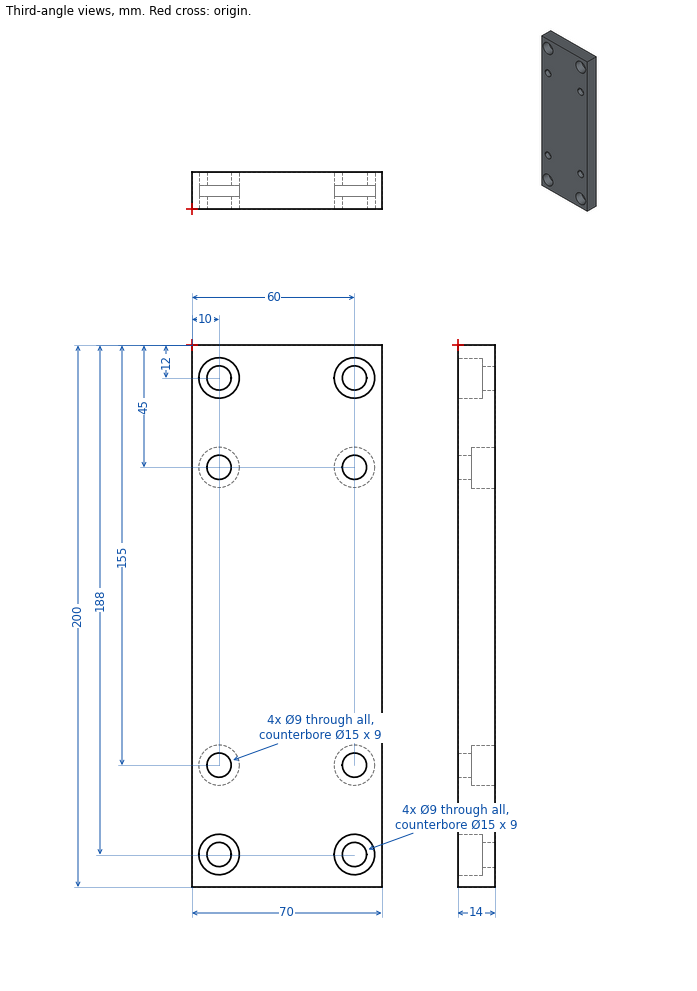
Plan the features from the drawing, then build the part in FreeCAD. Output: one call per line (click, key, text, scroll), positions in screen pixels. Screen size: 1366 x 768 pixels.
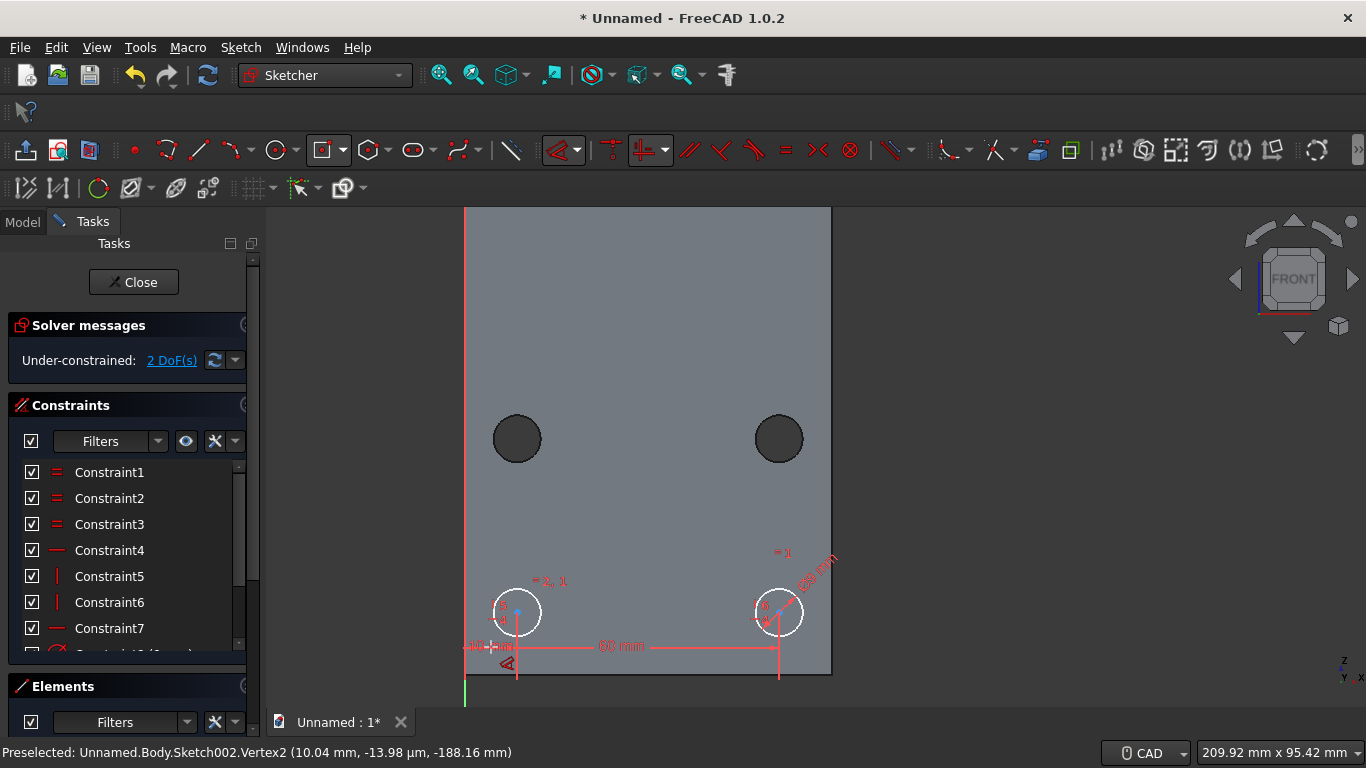
scroll(797, 598, down, 6)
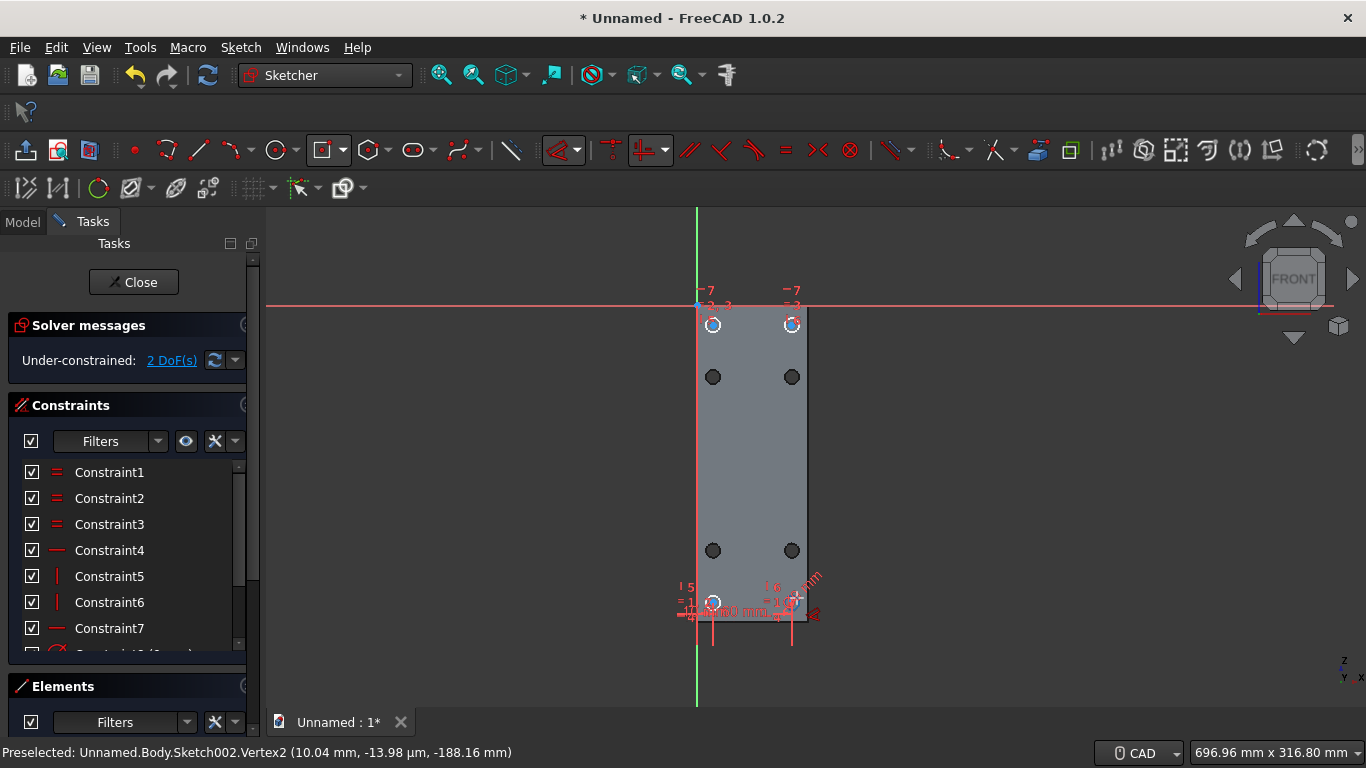
scroll(713, 325, up, 4)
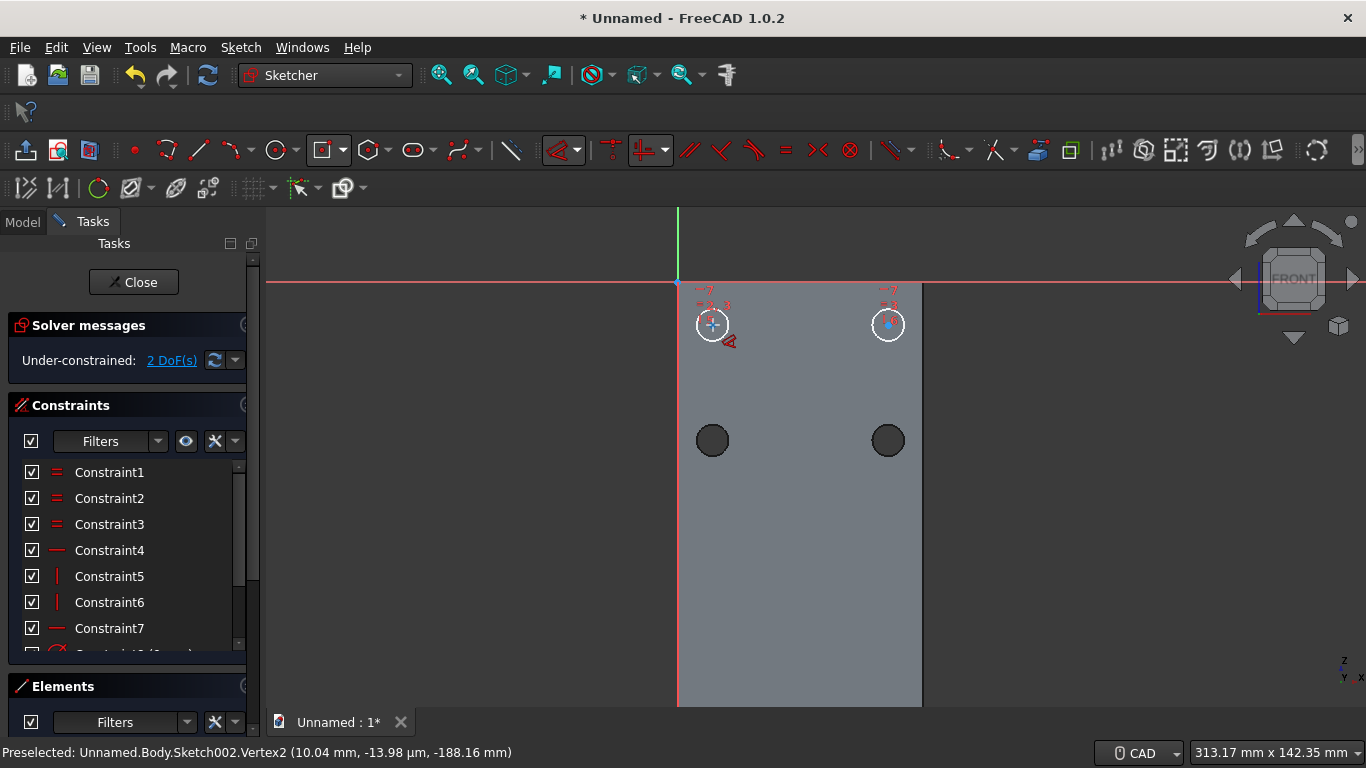
click(713, 325)
click(644, 304)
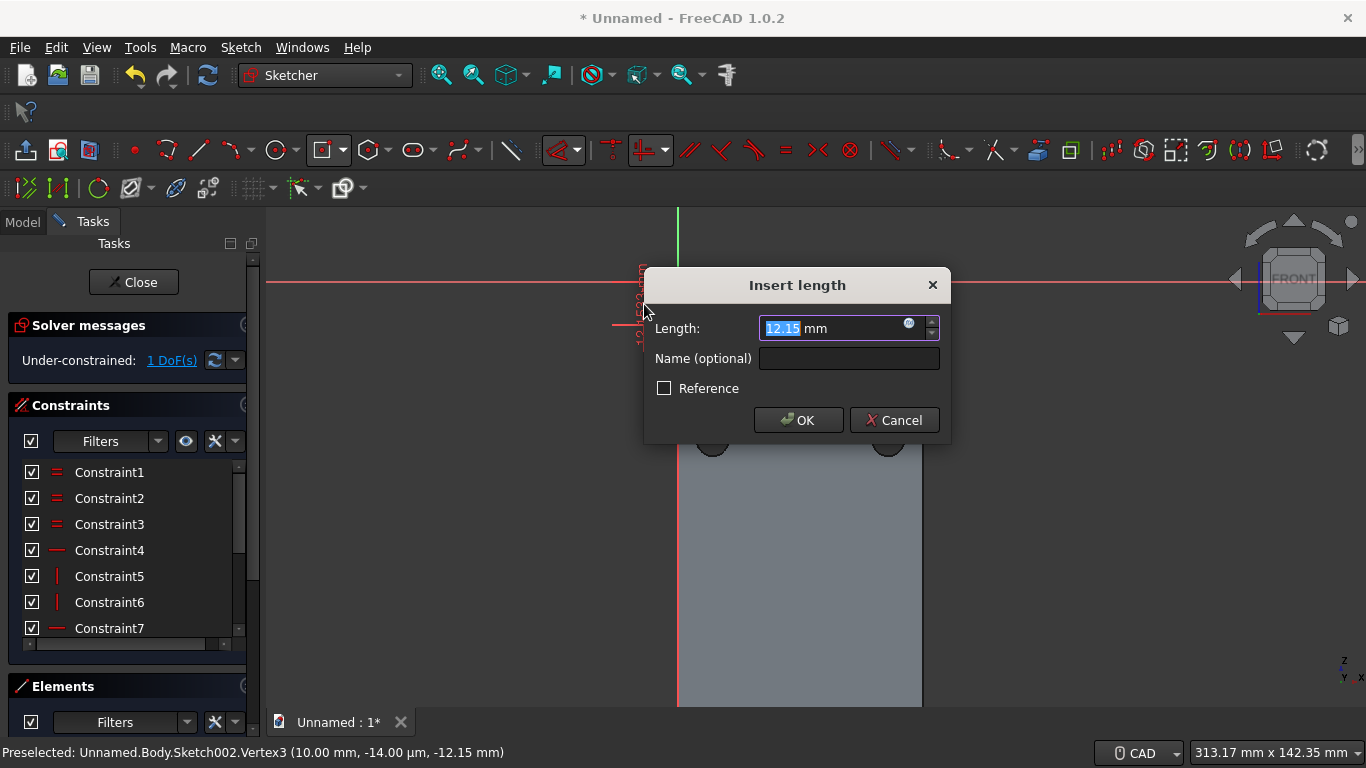
text(12)
key(Return)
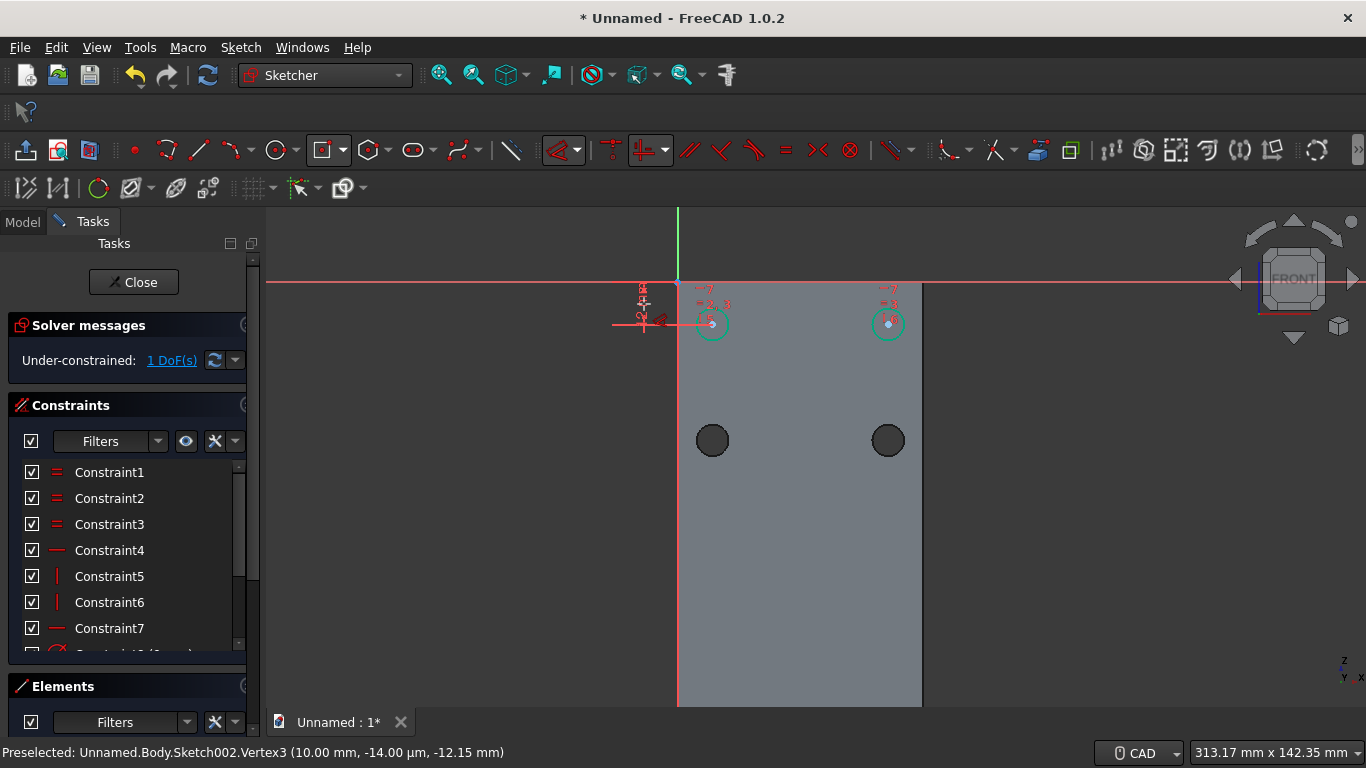
scroll(712, 324, down, 4)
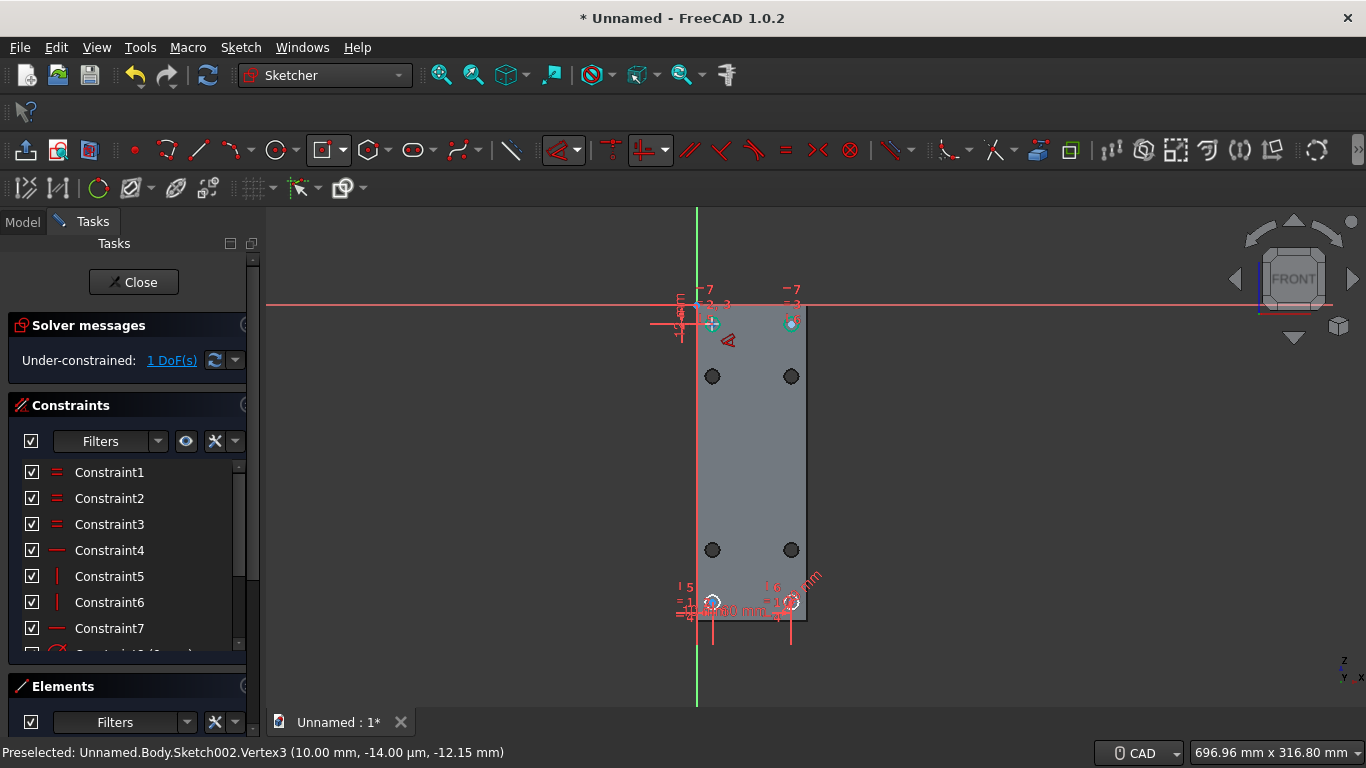
click(791, 602)
click(663, 454)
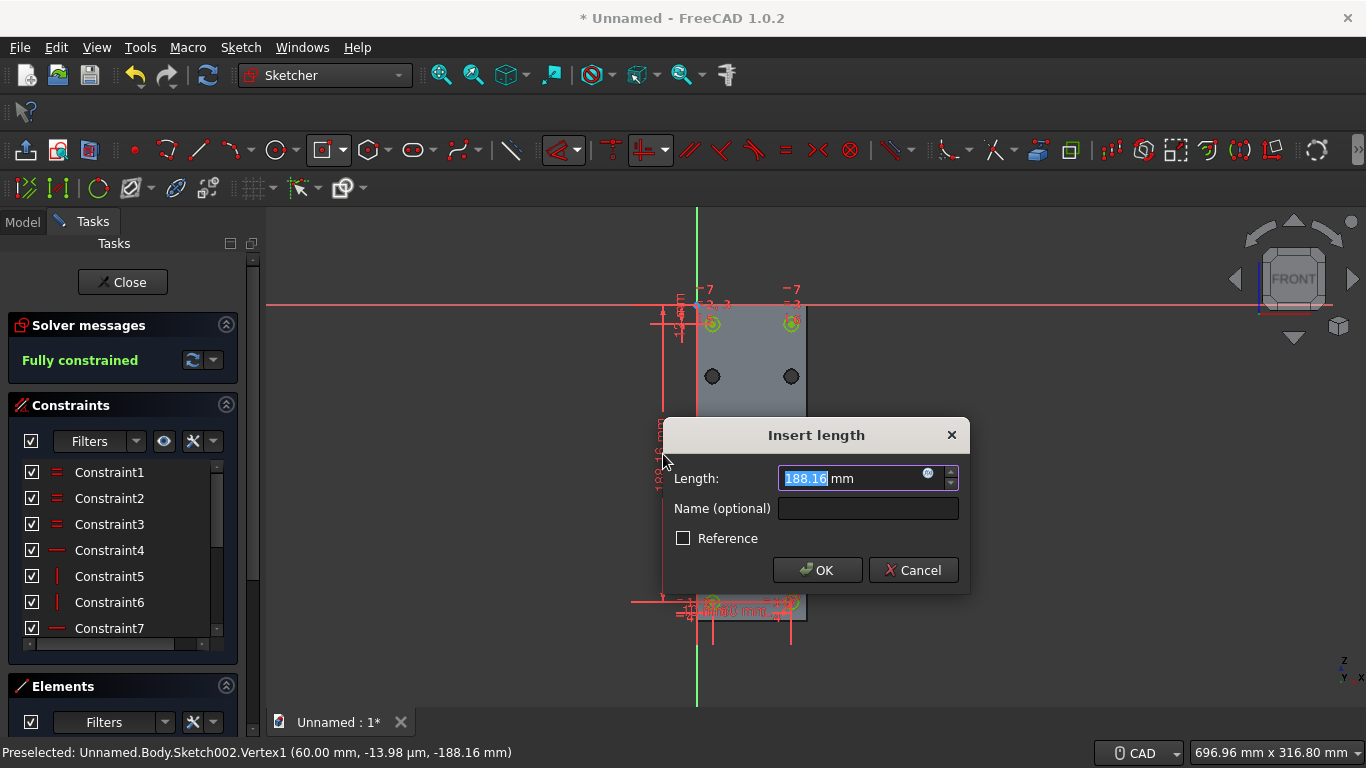
text(188)
key(Return)
key(Escape)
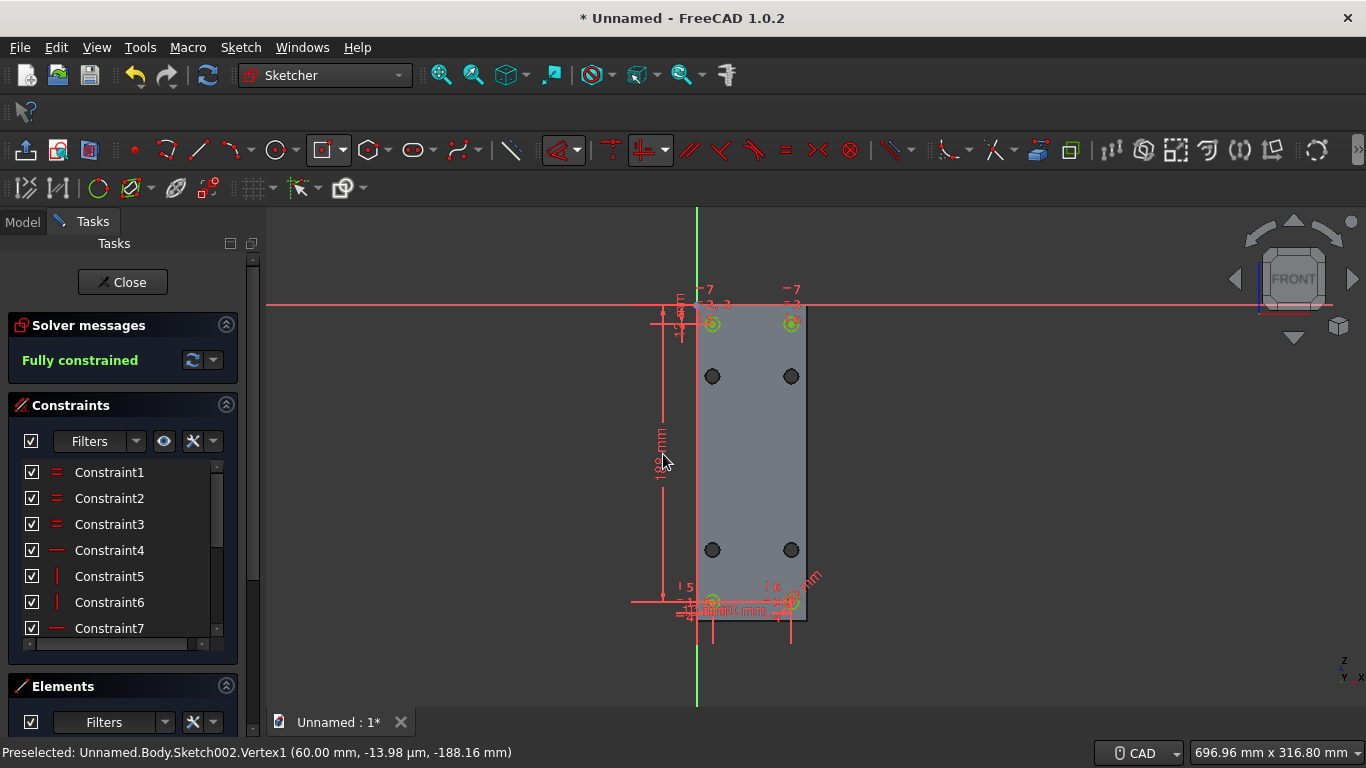
click(123, 282)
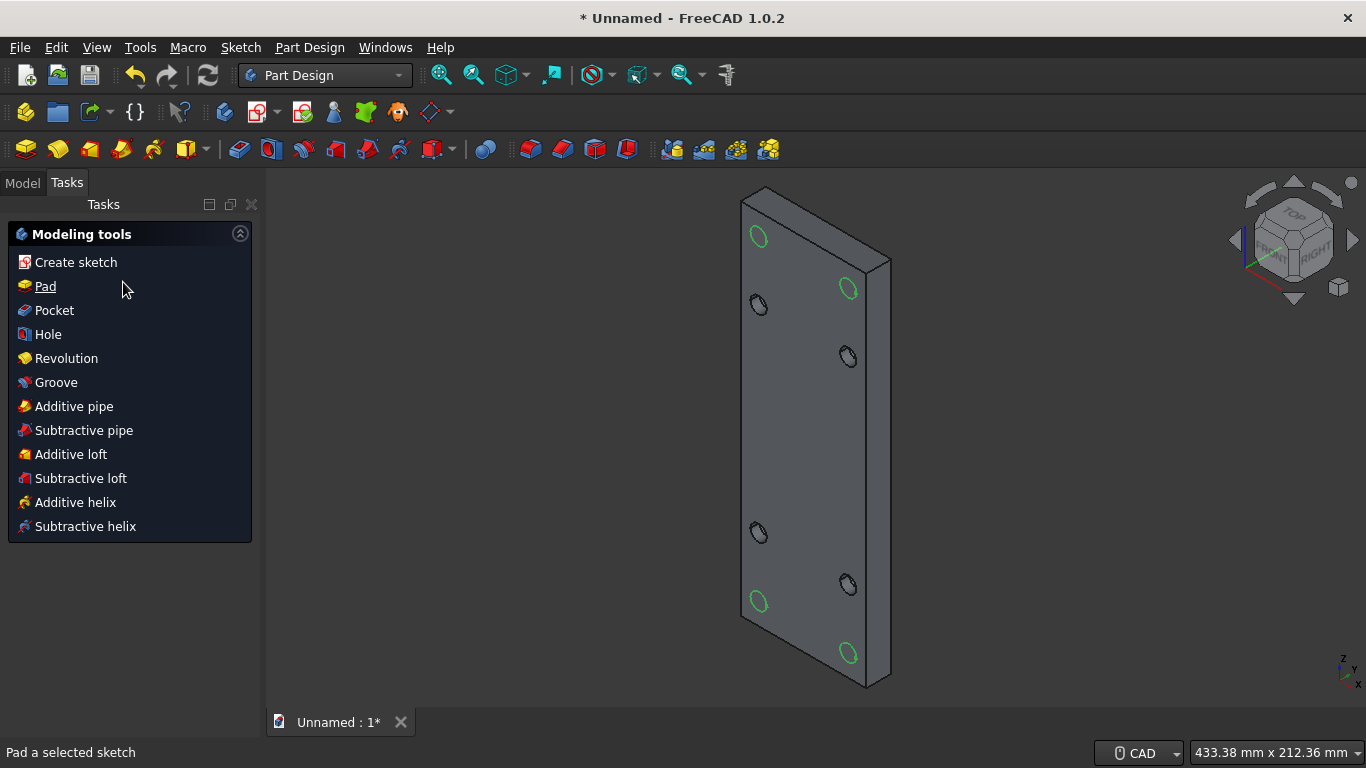
click(272, 150)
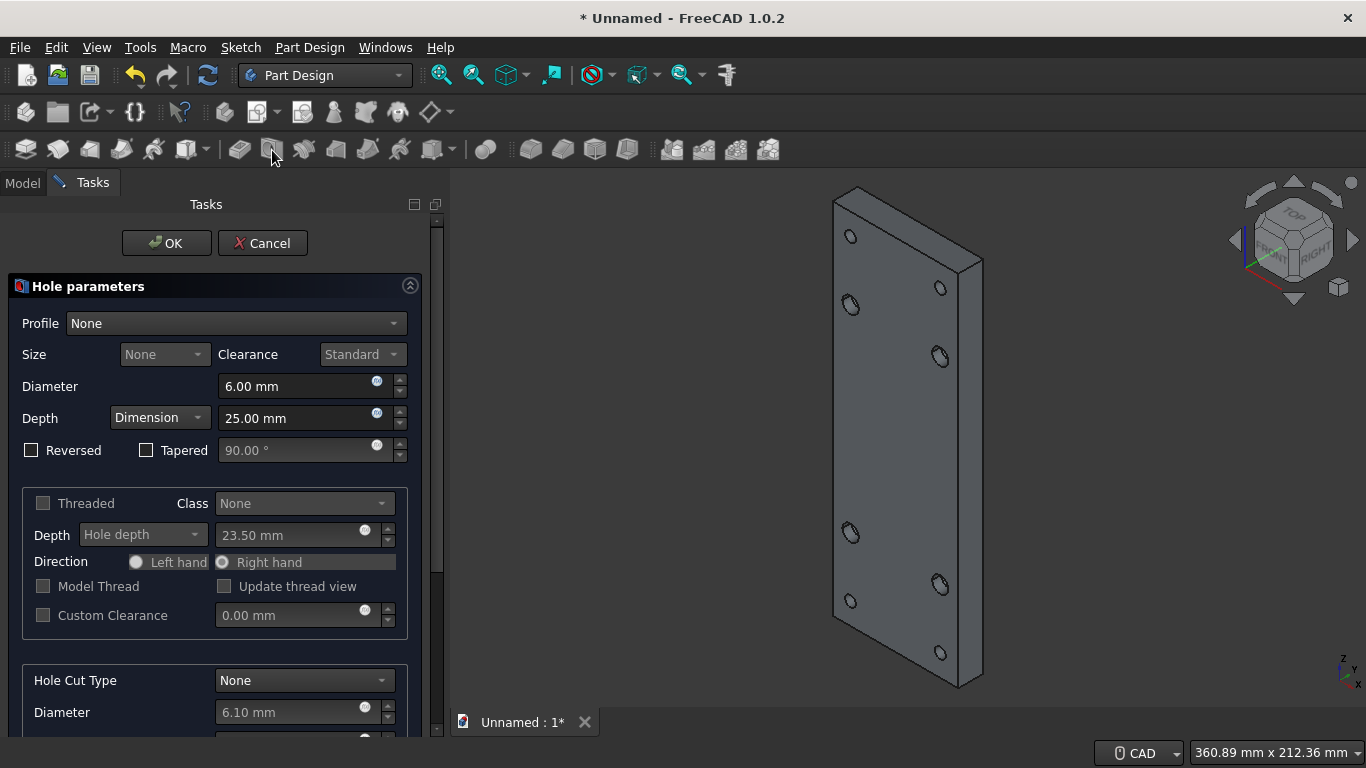
triple_click(305, 386)